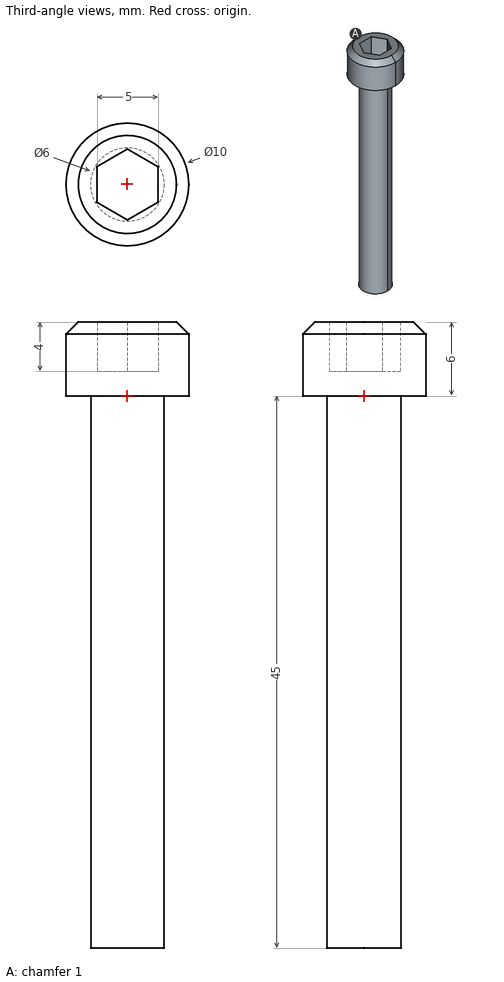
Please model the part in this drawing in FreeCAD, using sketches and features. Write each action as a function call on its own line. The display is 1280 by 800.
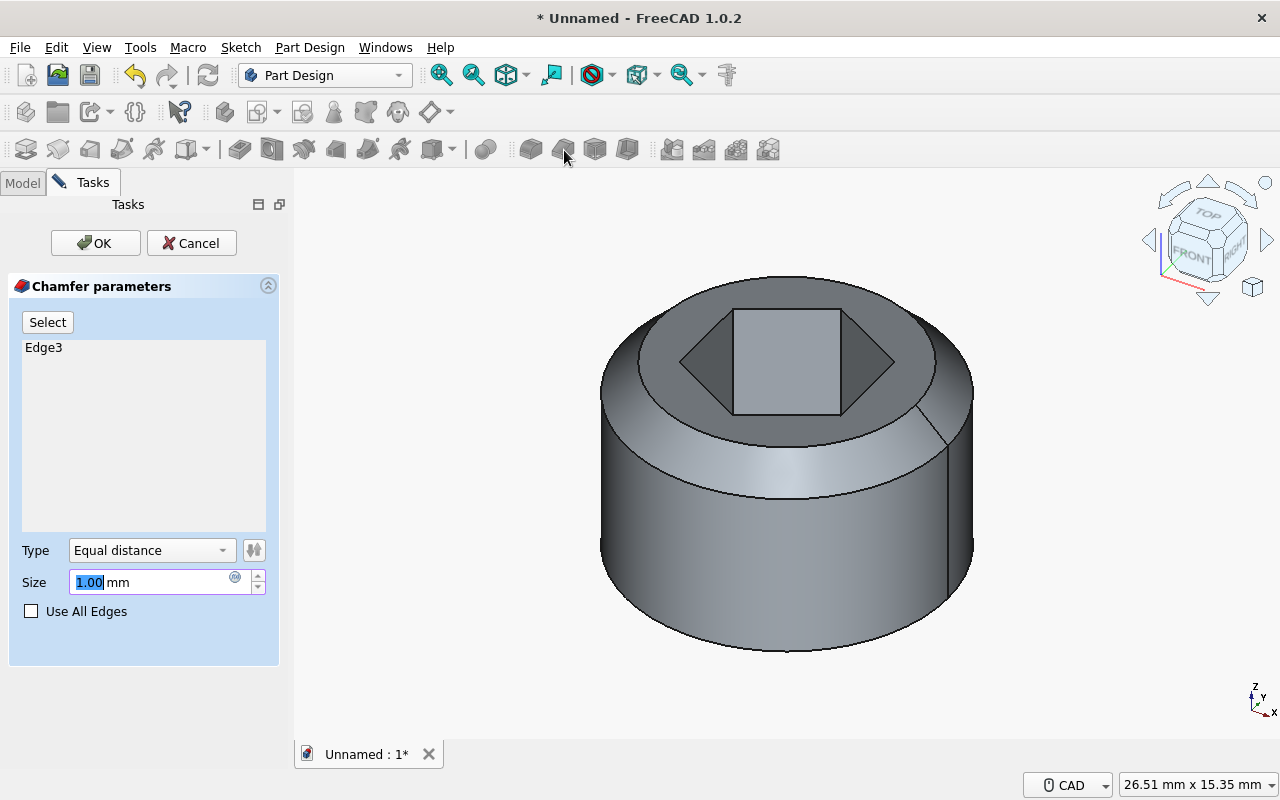
text(1)
key(Tab)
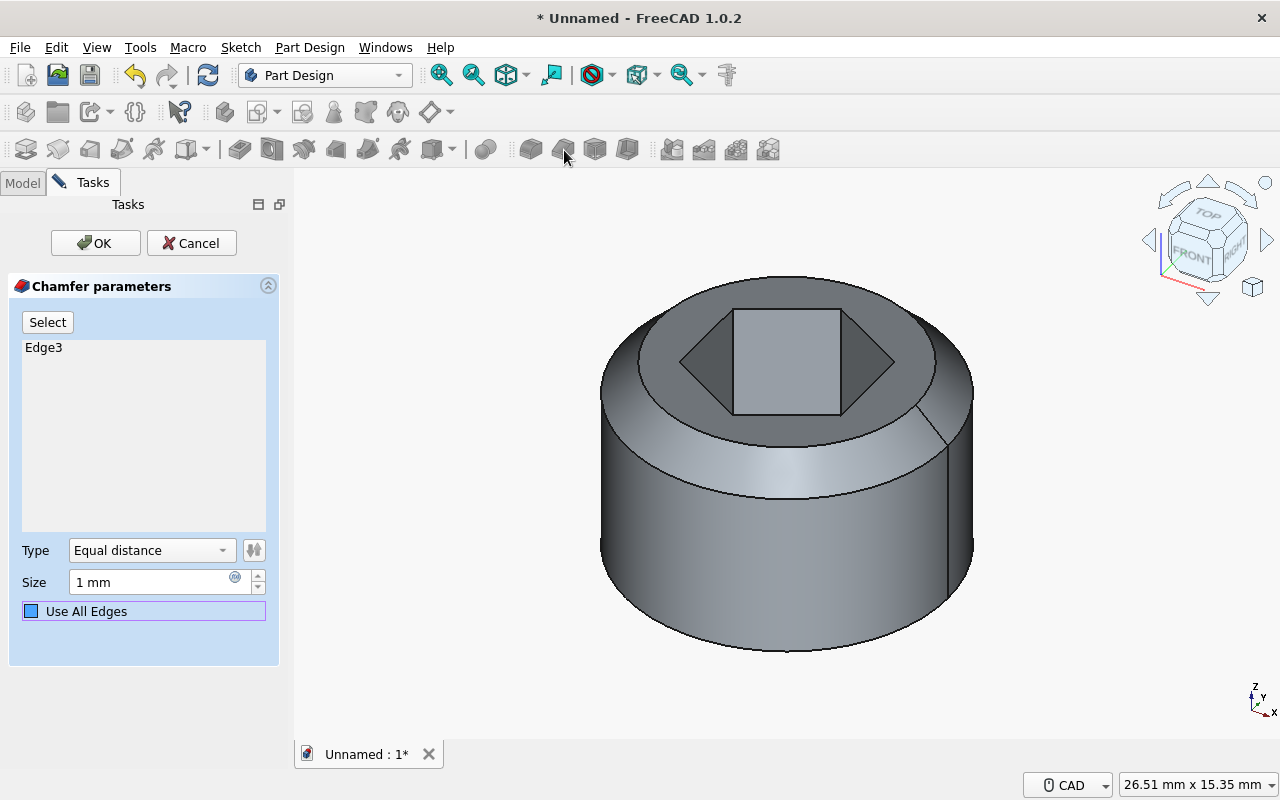
click(96, 243)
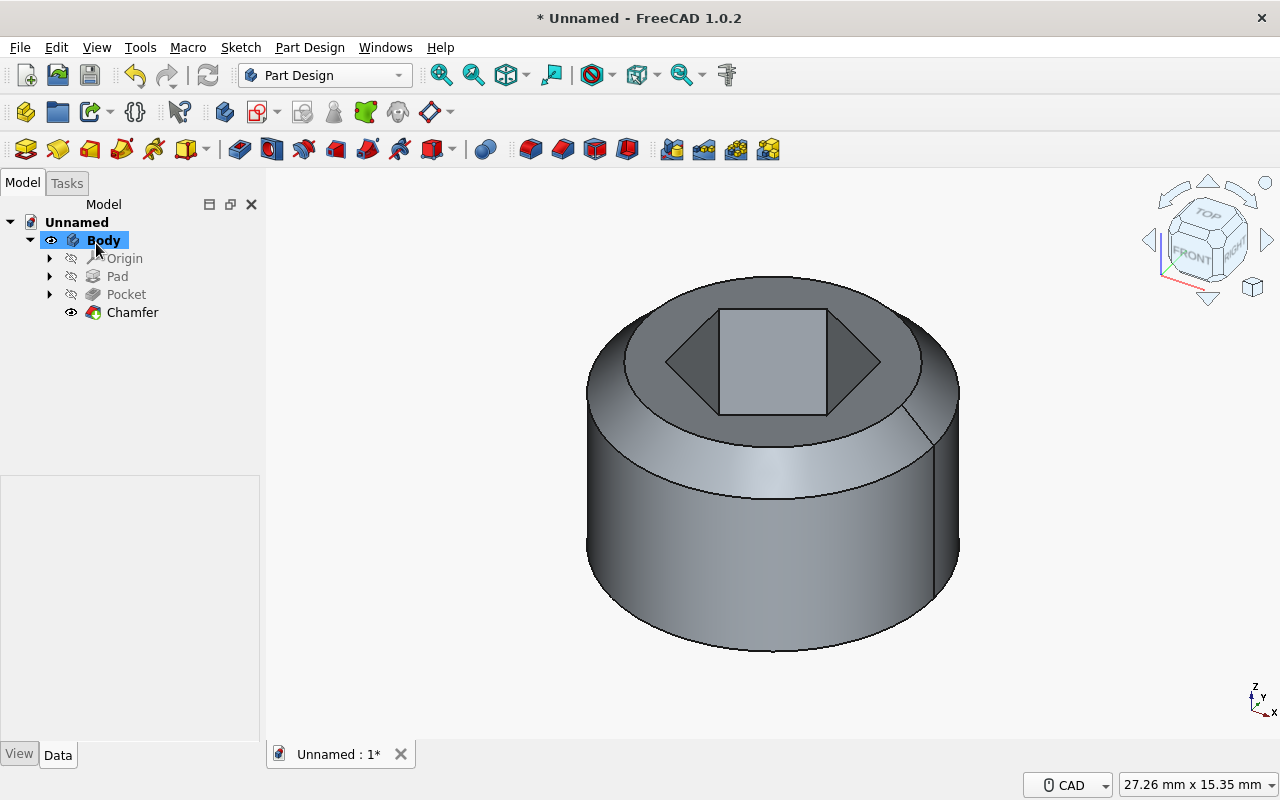
key(5)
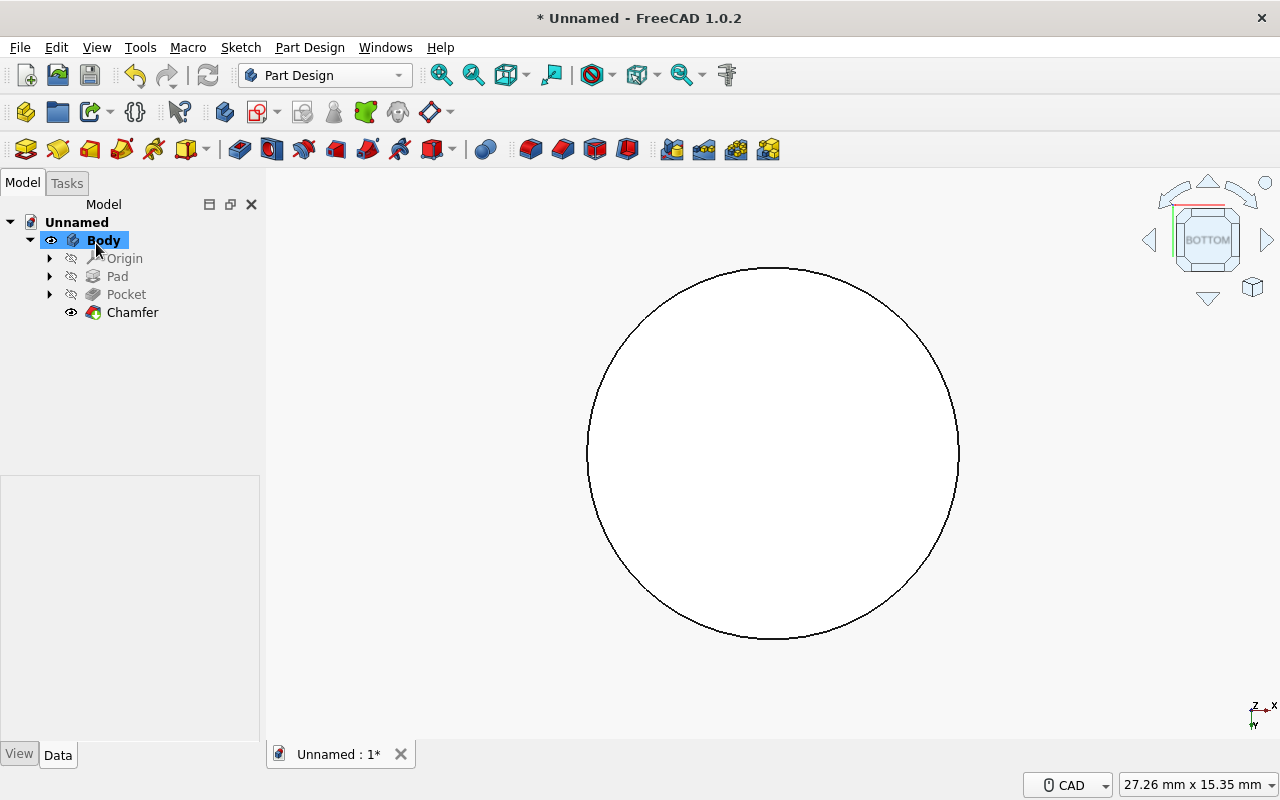
click(773, 453)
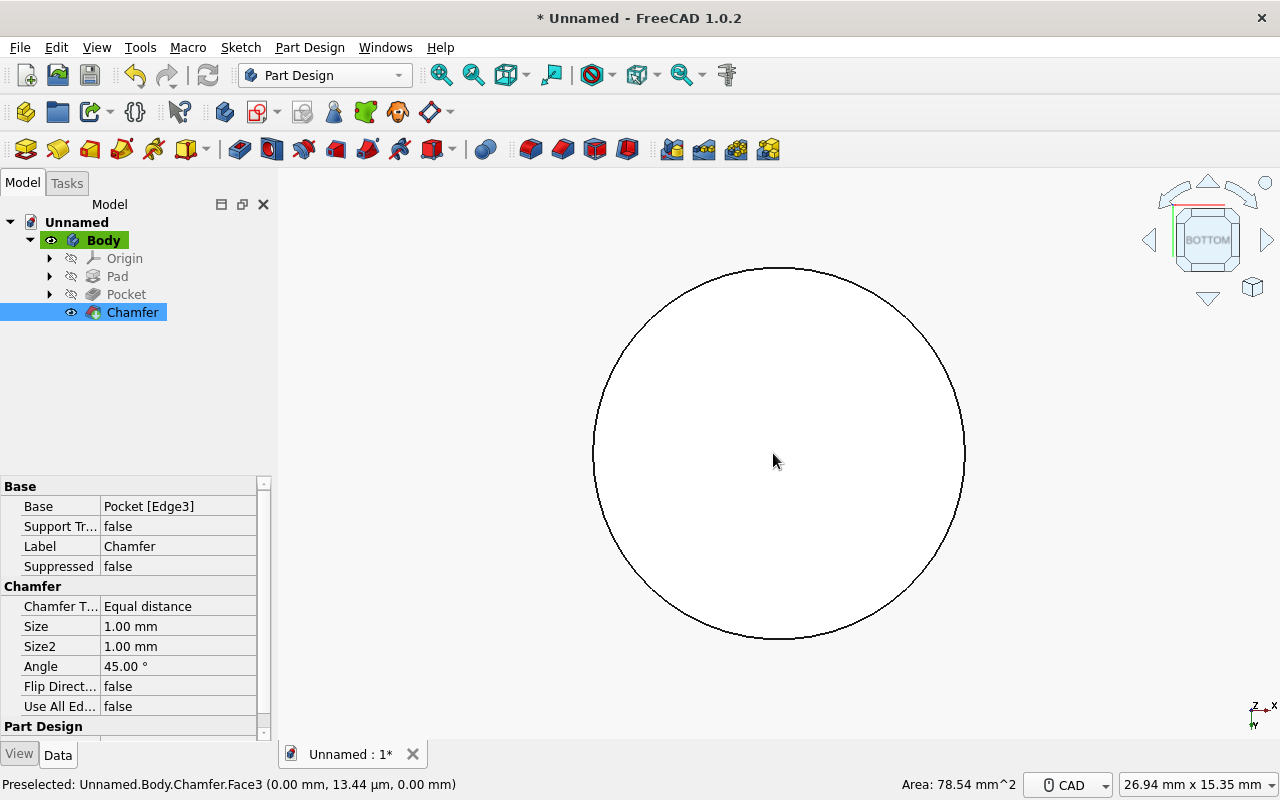
click(258, 112)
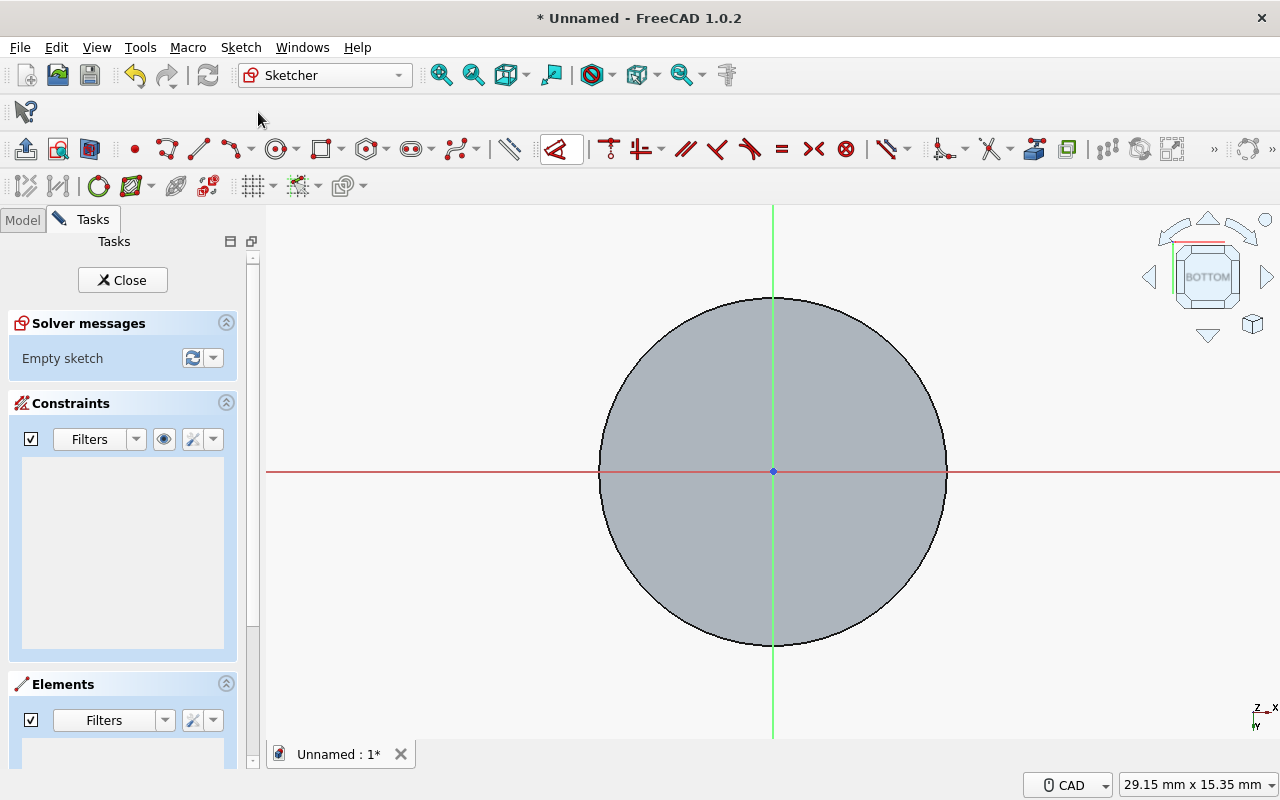
scroll(912, 472, up, 2)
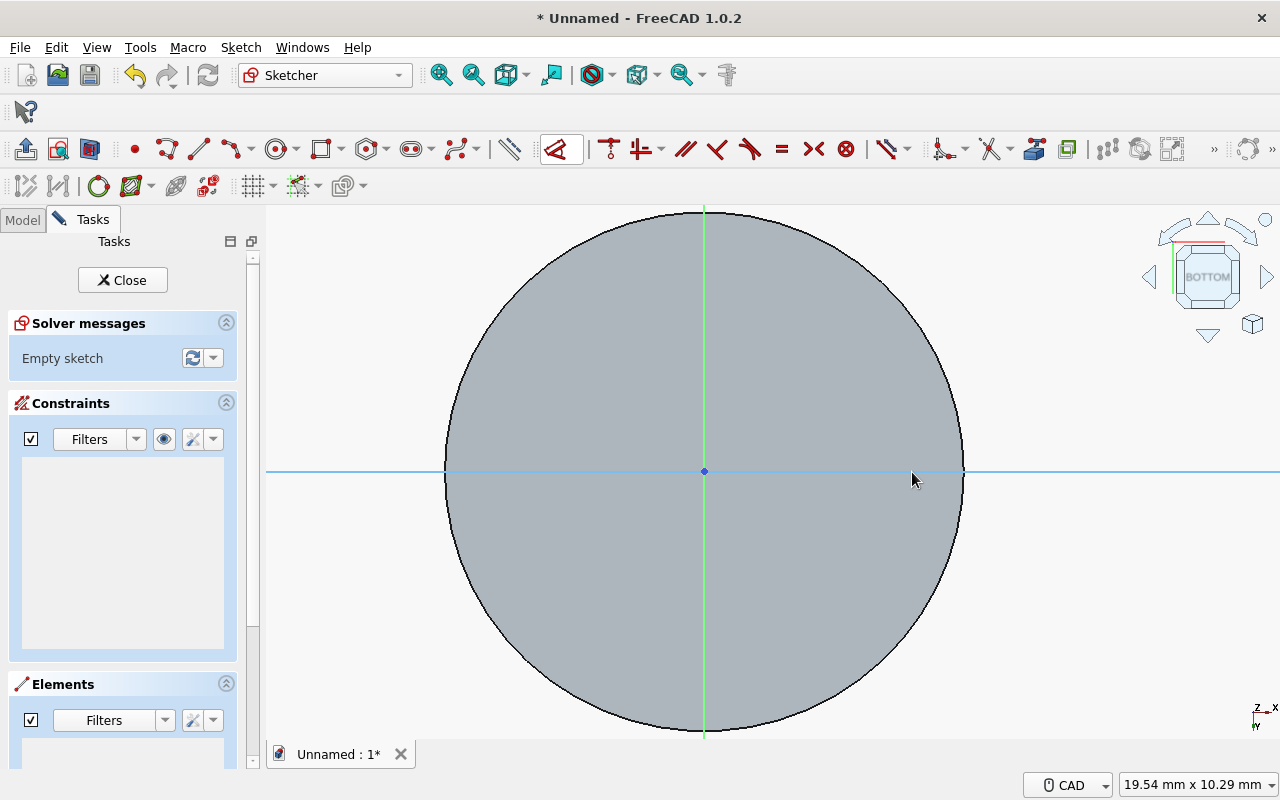
click(276, 150)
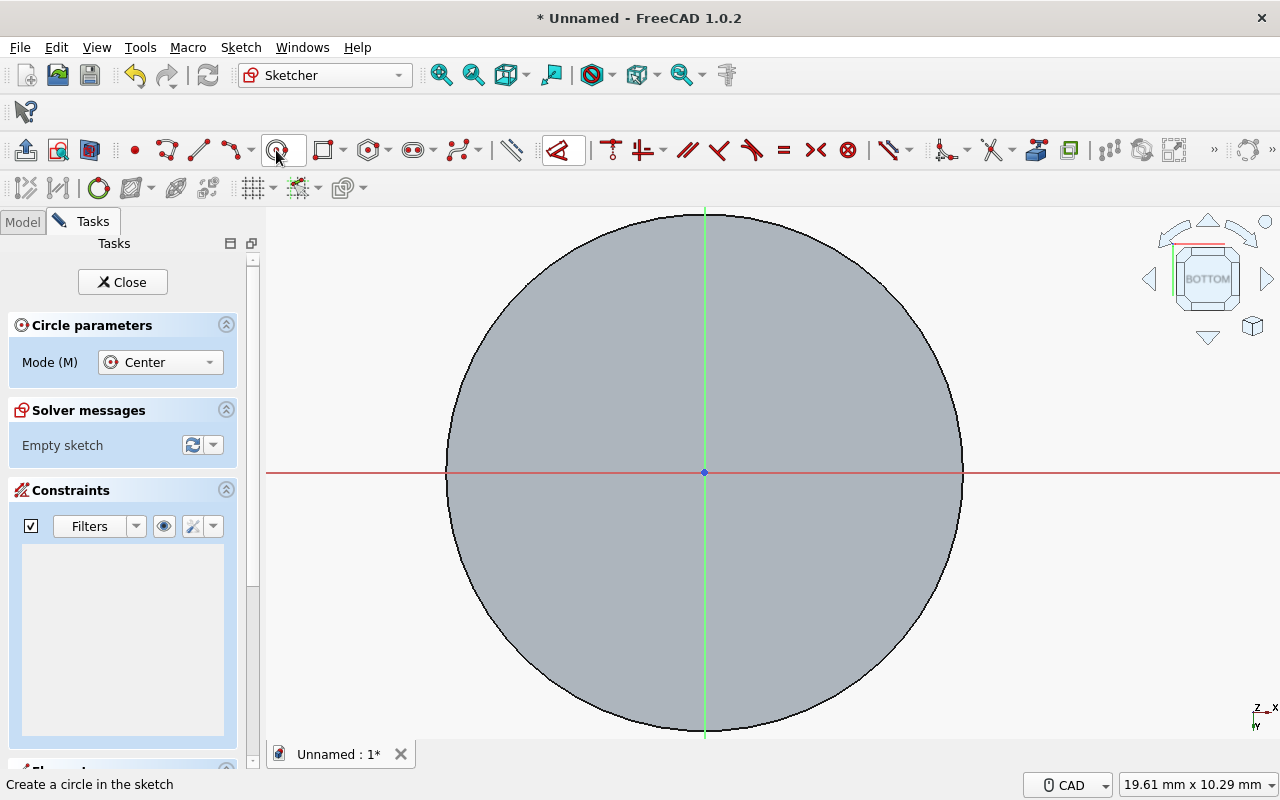
click(705, 473)
move(814, 363)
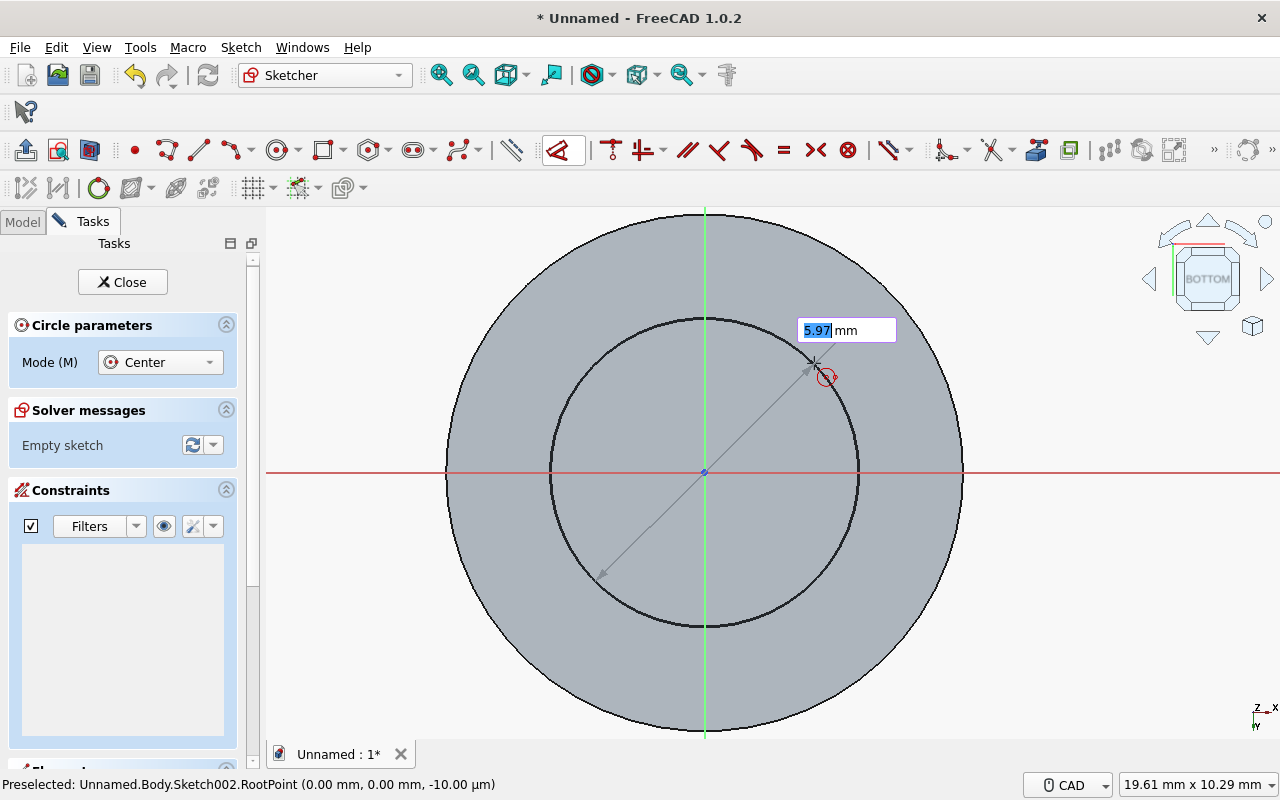
text(6)
key(Return)
key(Escape)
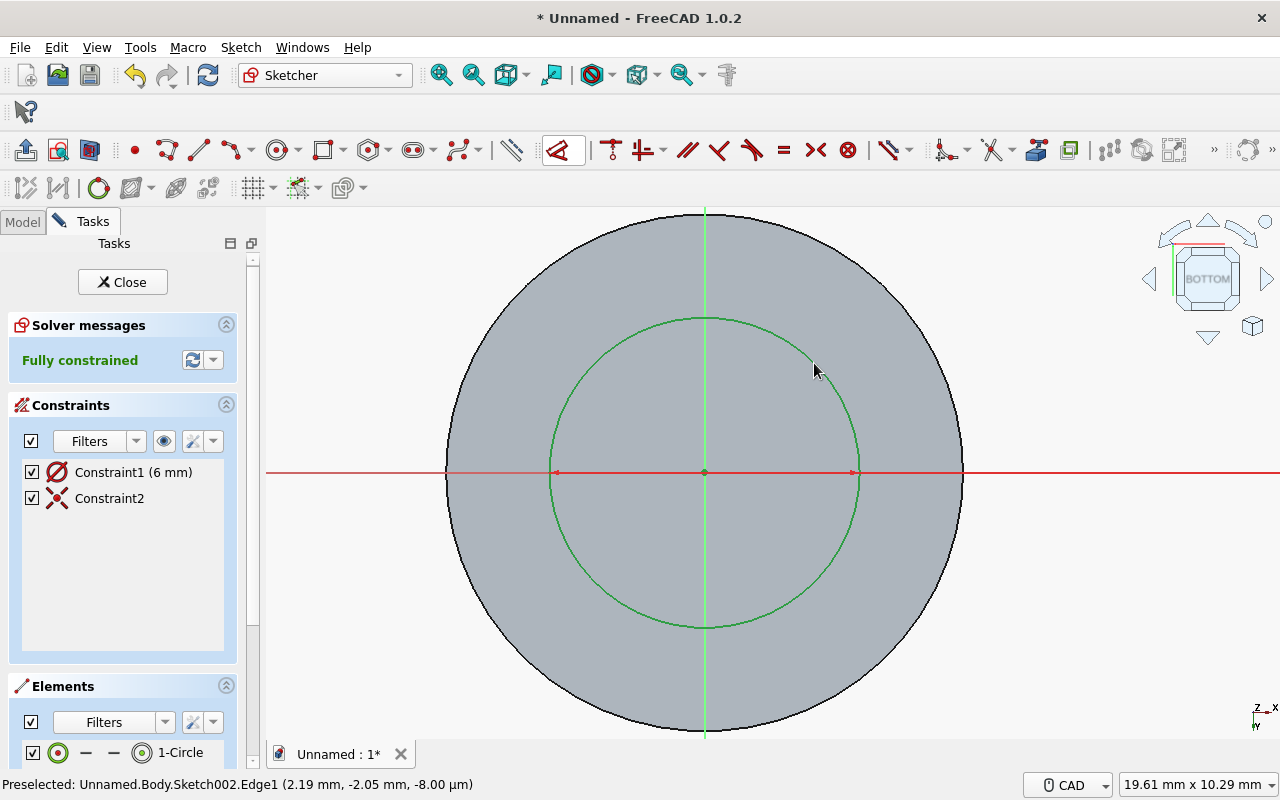
click(123, 282)